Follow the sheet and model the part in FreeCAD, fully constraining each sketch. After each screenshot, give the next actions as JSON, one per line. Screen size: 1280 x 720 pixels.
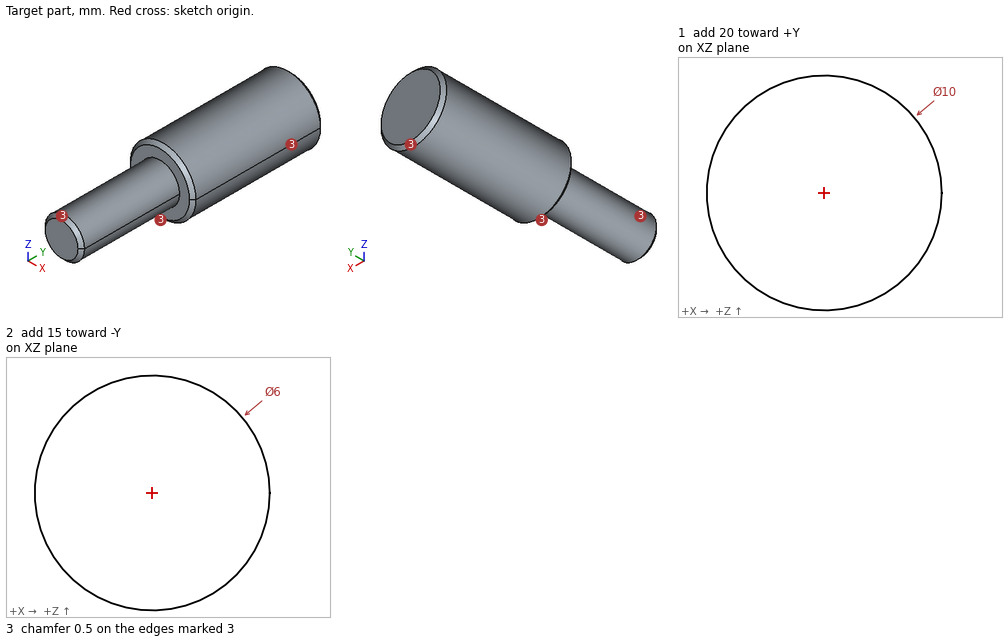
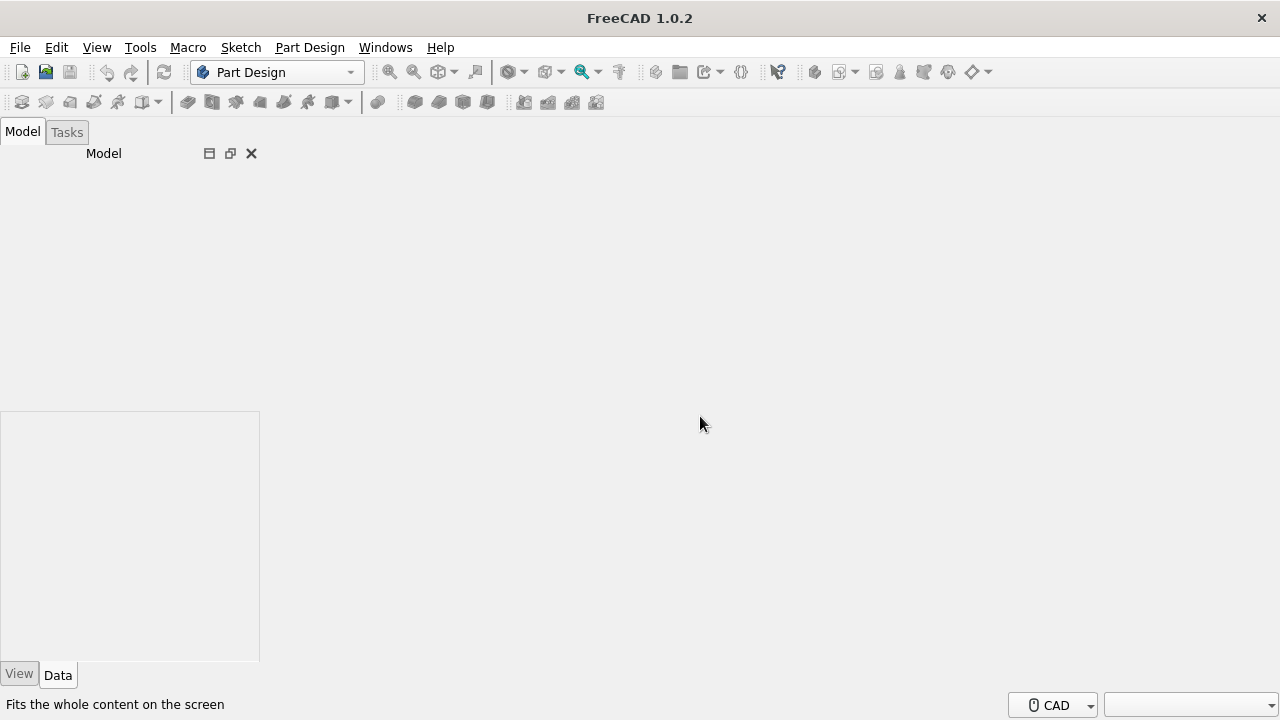
{"action": "left_click", "coordinate": [22, 72]}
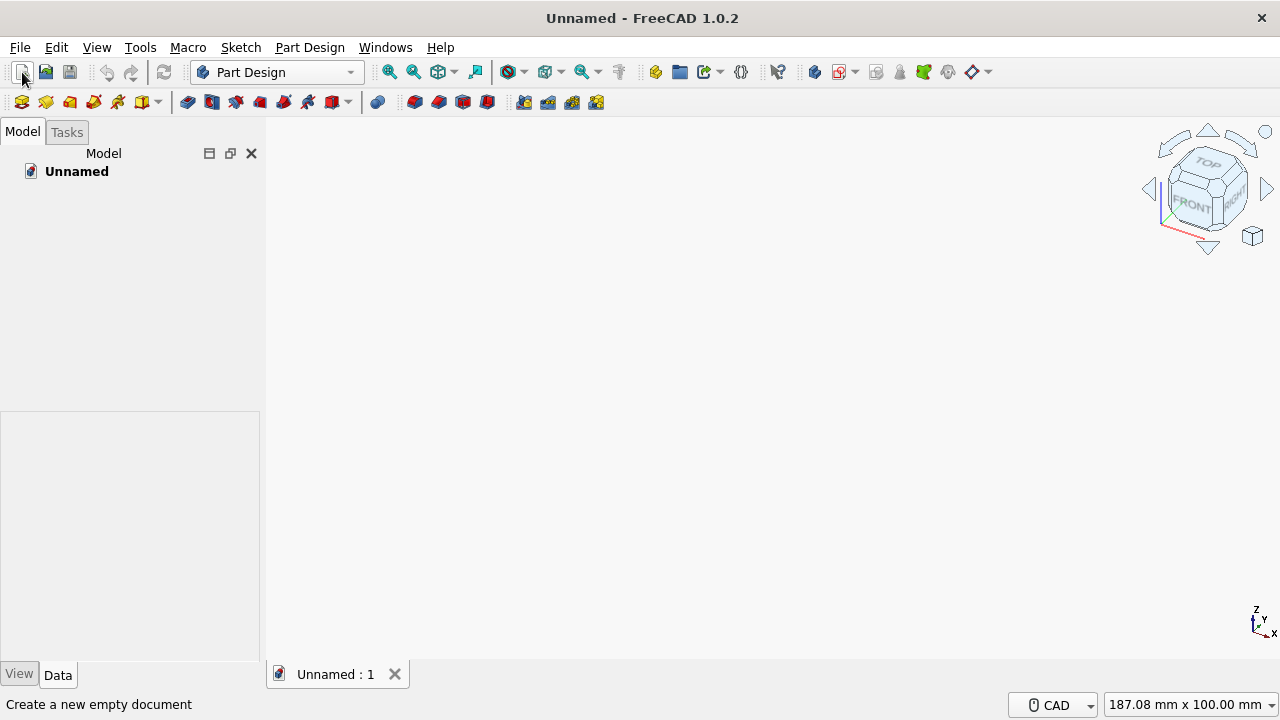
{"action": "left_click", "coordinate": [840, 72]}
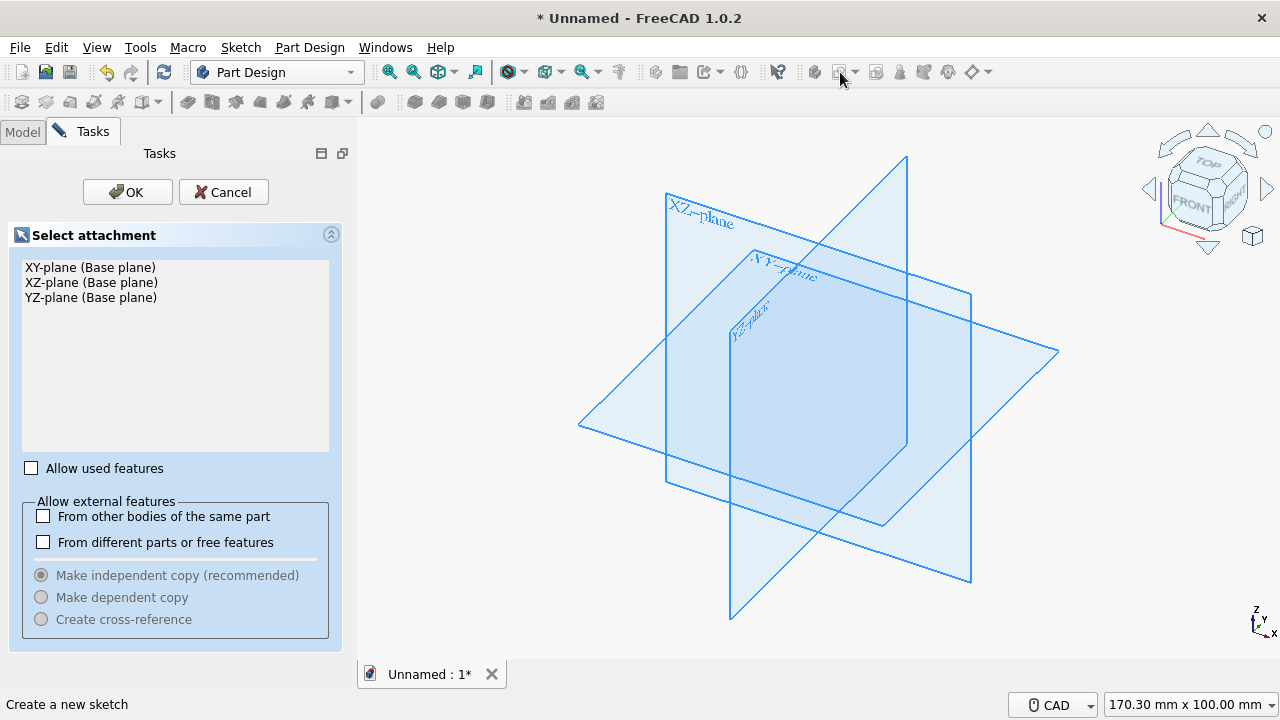
{"action": "left_click", "coordinate": [82, 282]}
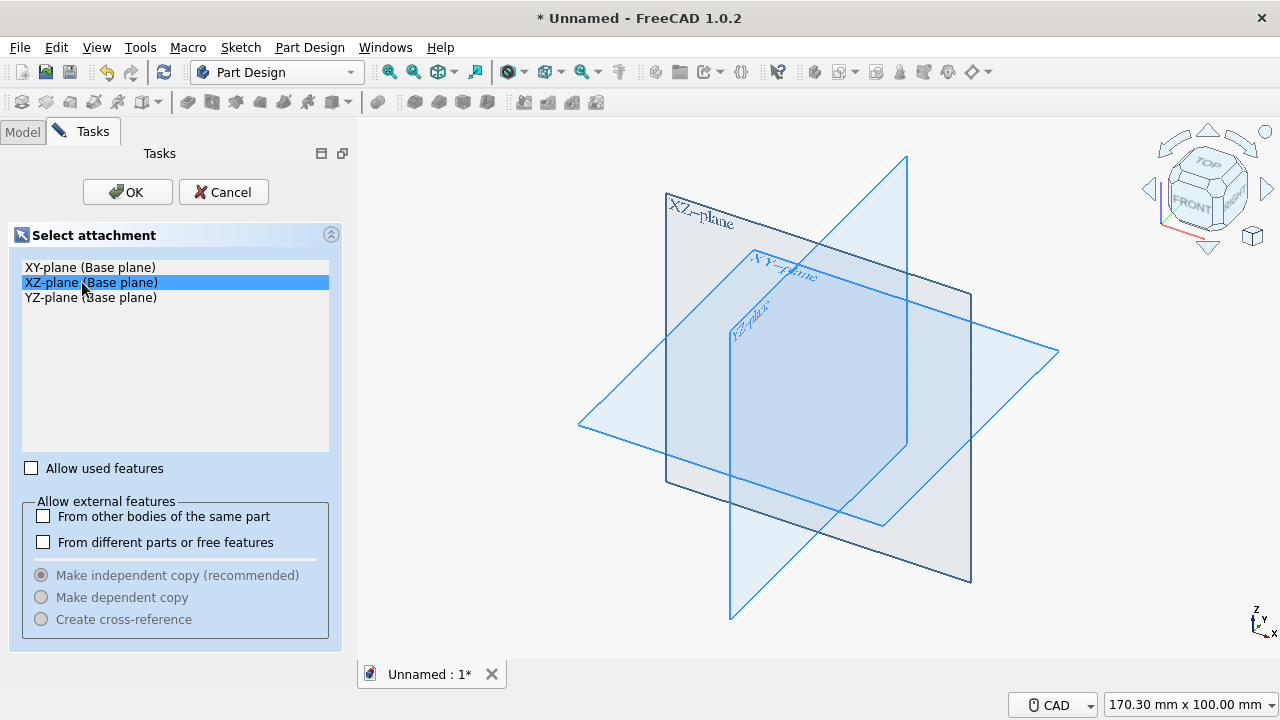
{"action": "left_click", "coordinate": [128, 192]}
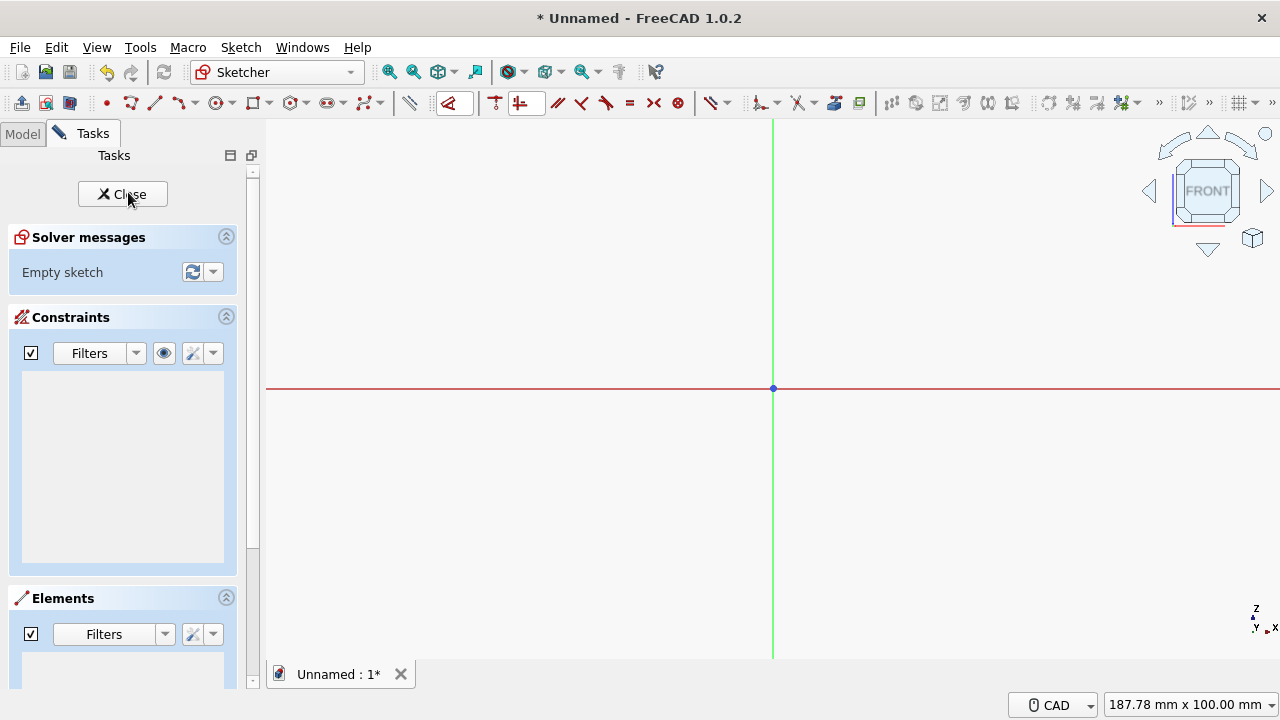
{"action": "scroll", "coordinate": [787, 389], "scroll_direction": "up", "scroll_amount": 9}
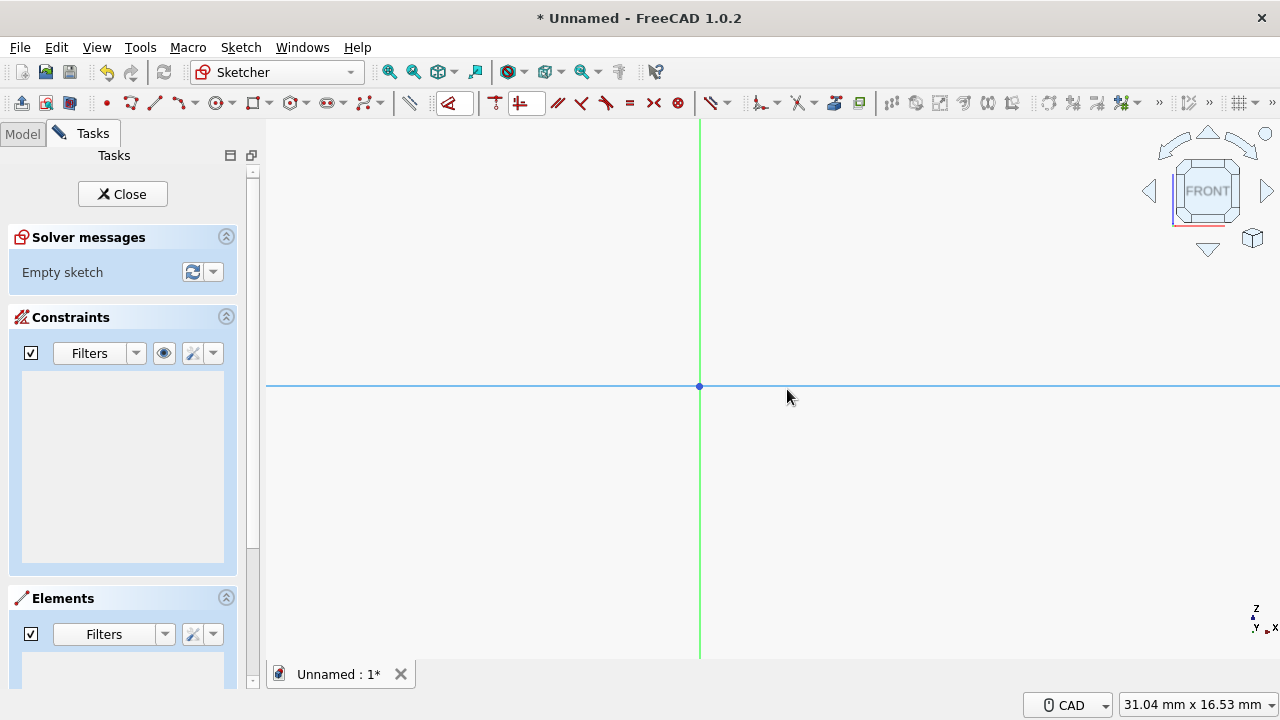
{"action": "left_click", "coordinate": [216, 104]}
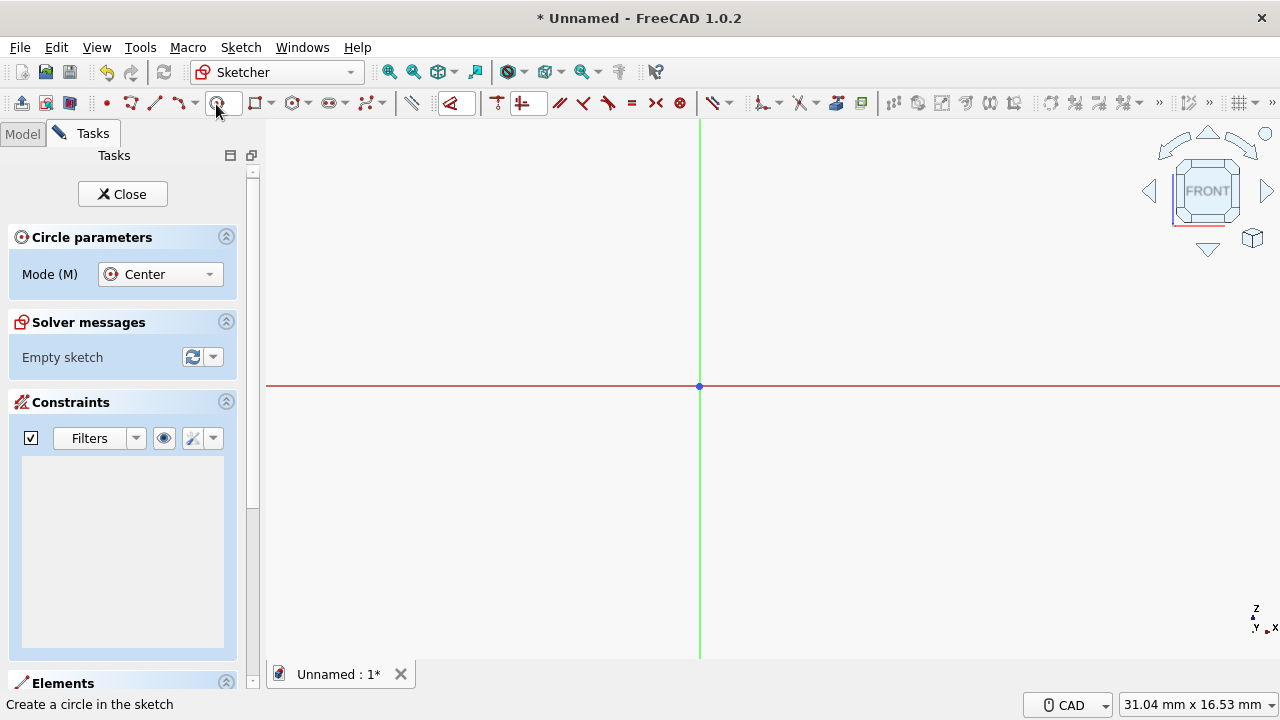
{"action": "left_click", "coordinate": [700, 386]}
{"action": "left_click", "coordinate": [815, 271]}
{"action": "key", "text": "Escape"}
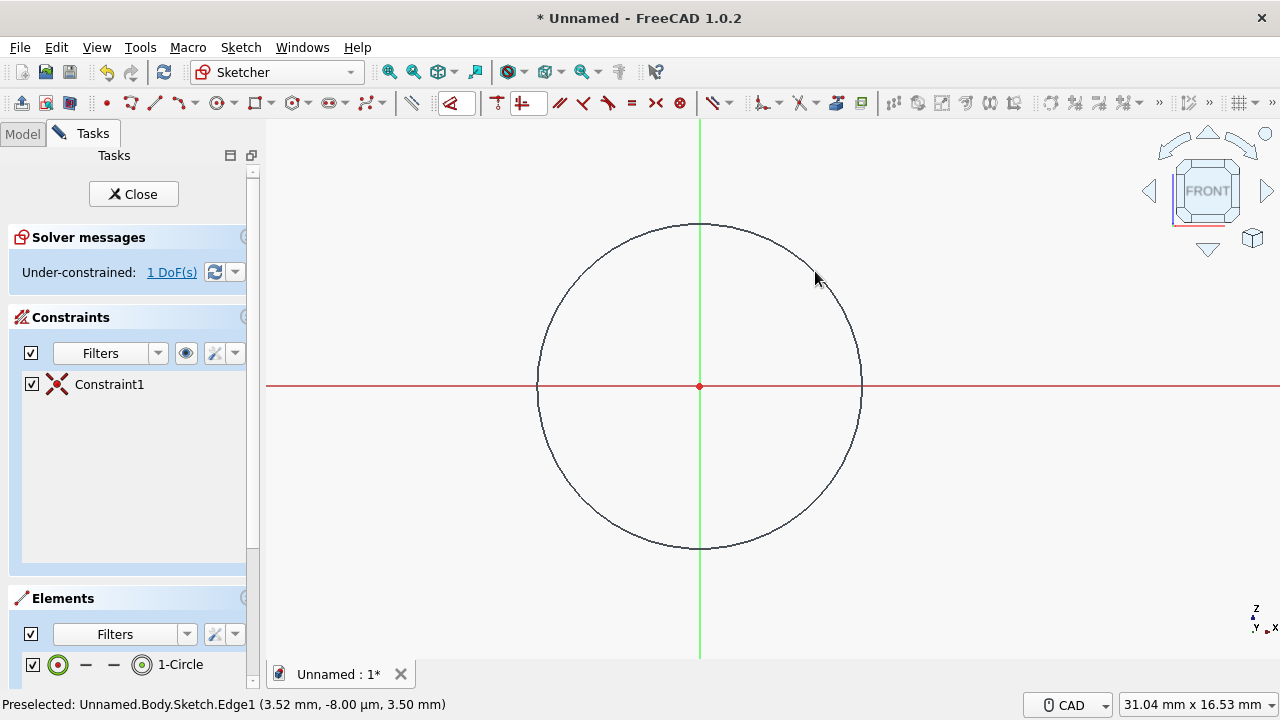
{"action": "left_click", "coordinate": [450, 104]}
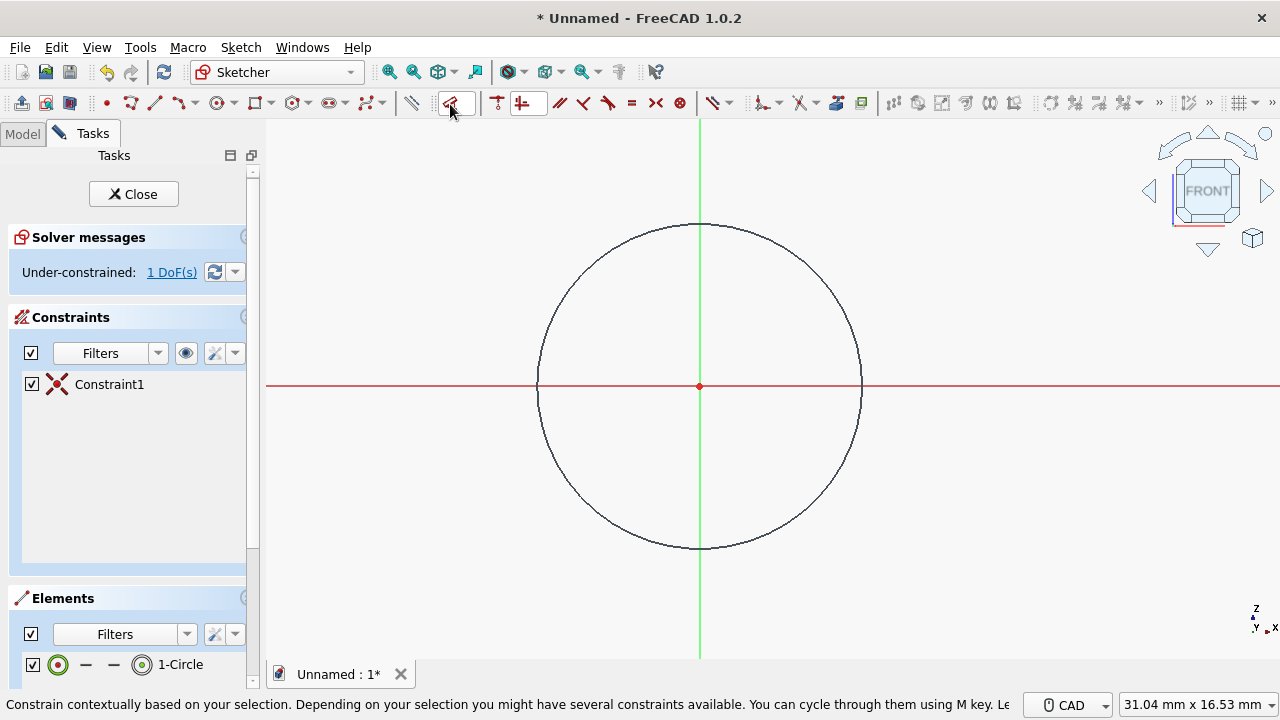
{"action": "left_click", "coordinate": [814, 271]}
{"action": "left_click", "coordinate": [837, 248]}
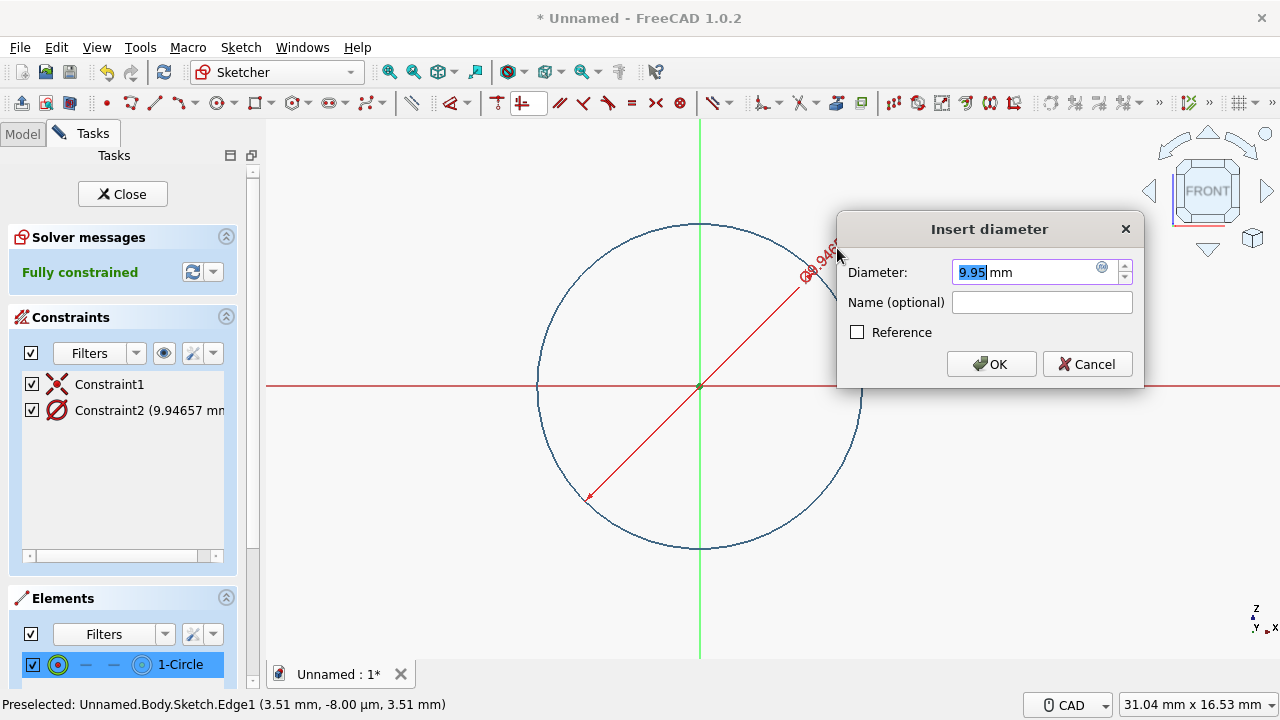
{"action": "type", "text": "10"}
{"action": "key", "text": "Return"}
{"action": "key", "text": "Escape"}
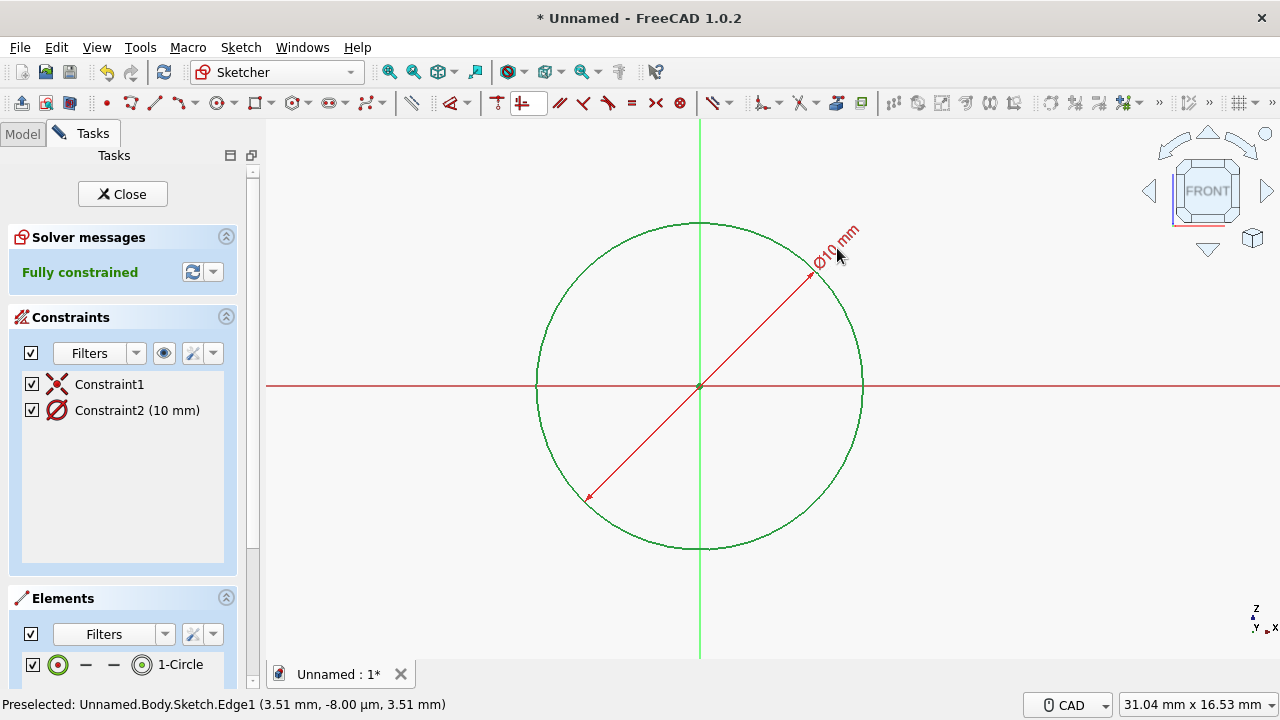
{"action": "left_click", "coordinate": [123, 194]}